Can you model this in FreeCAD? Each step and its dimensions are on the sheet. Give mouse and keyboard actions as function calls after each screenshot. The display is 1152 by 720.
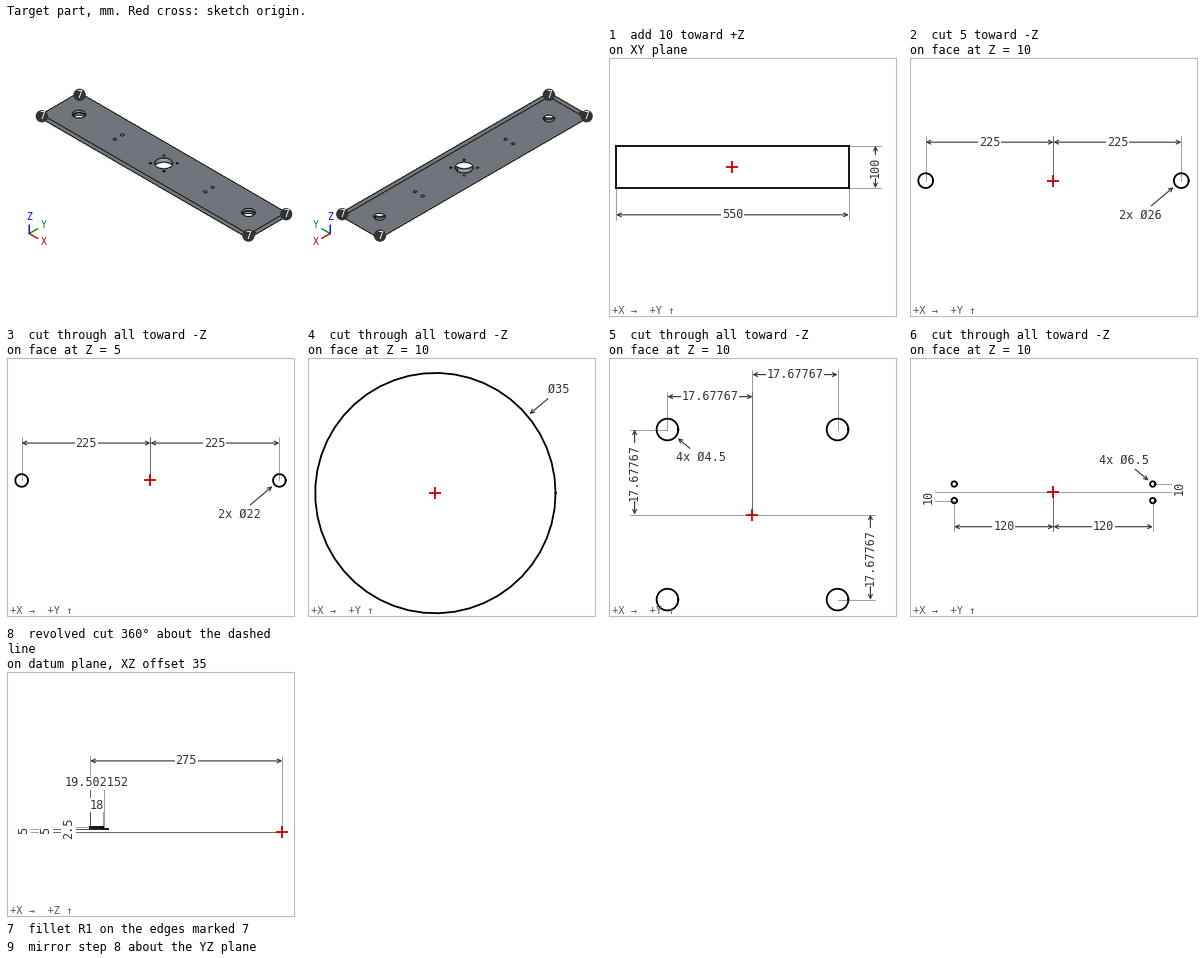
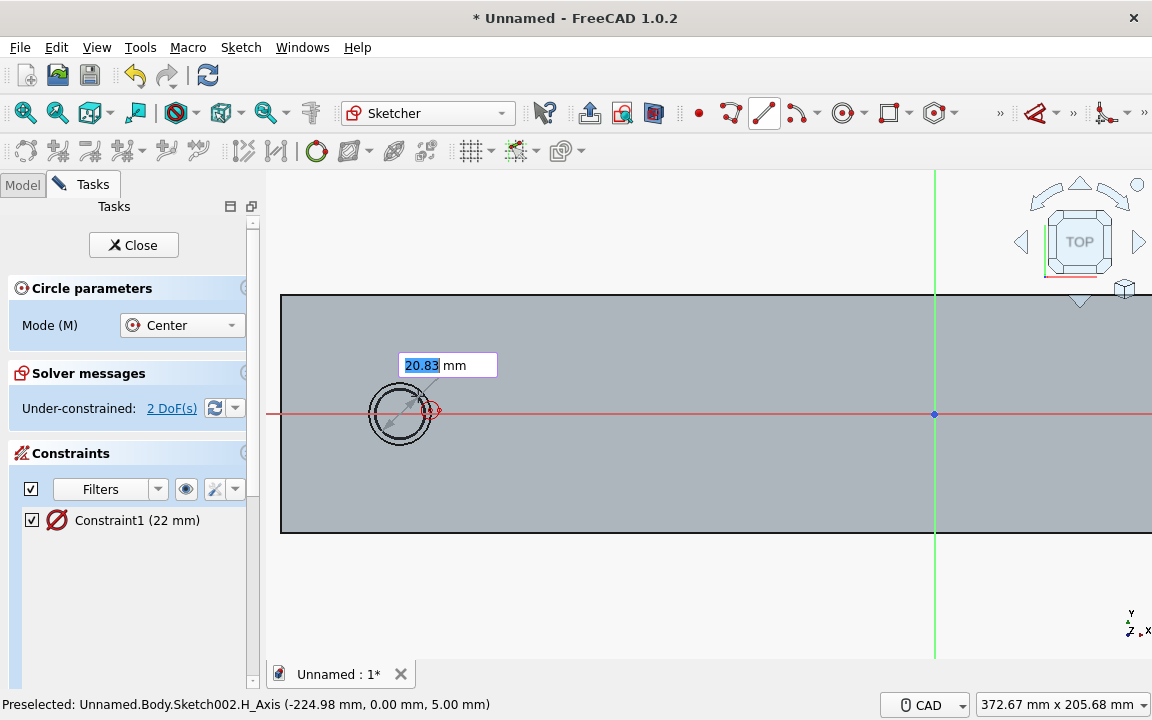
text(22)
key(Return)
key(Escape)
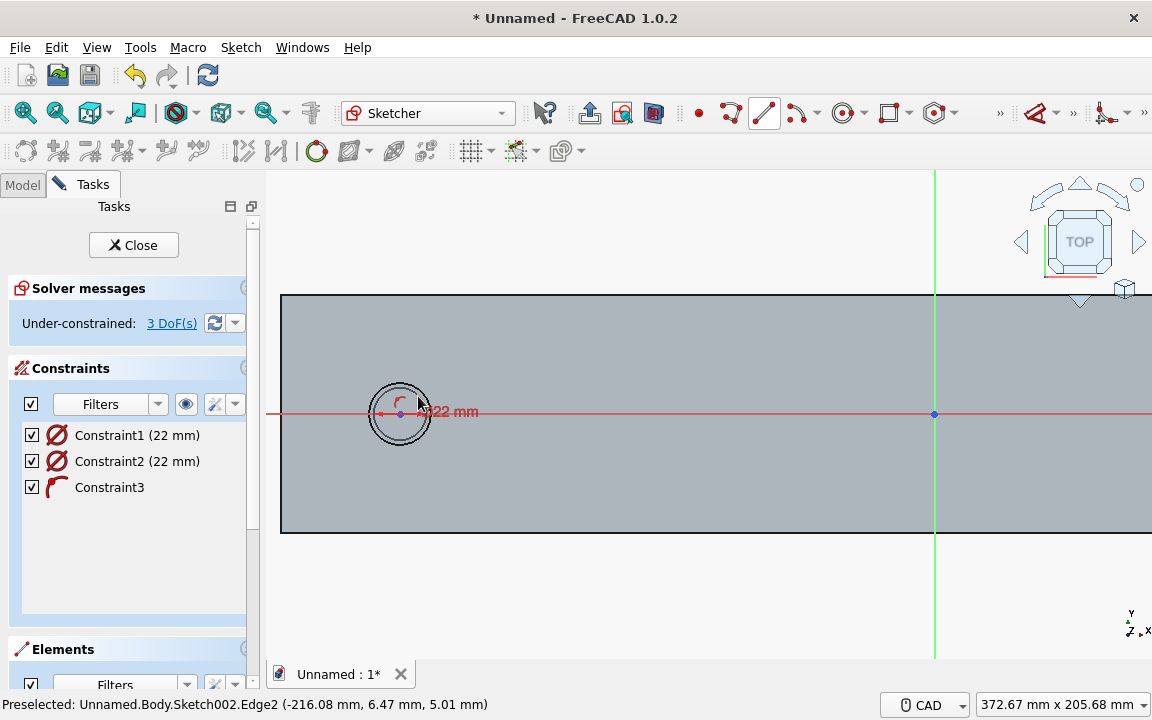
scroll(400, 415, down, 4)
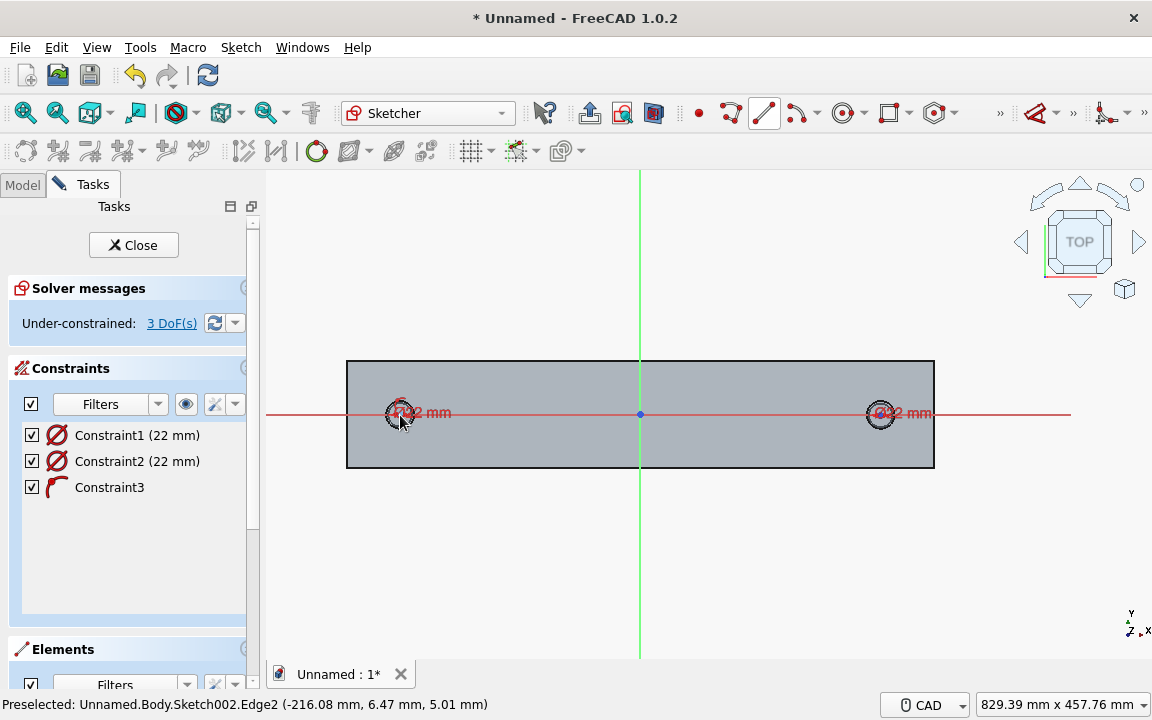
click(881, 415)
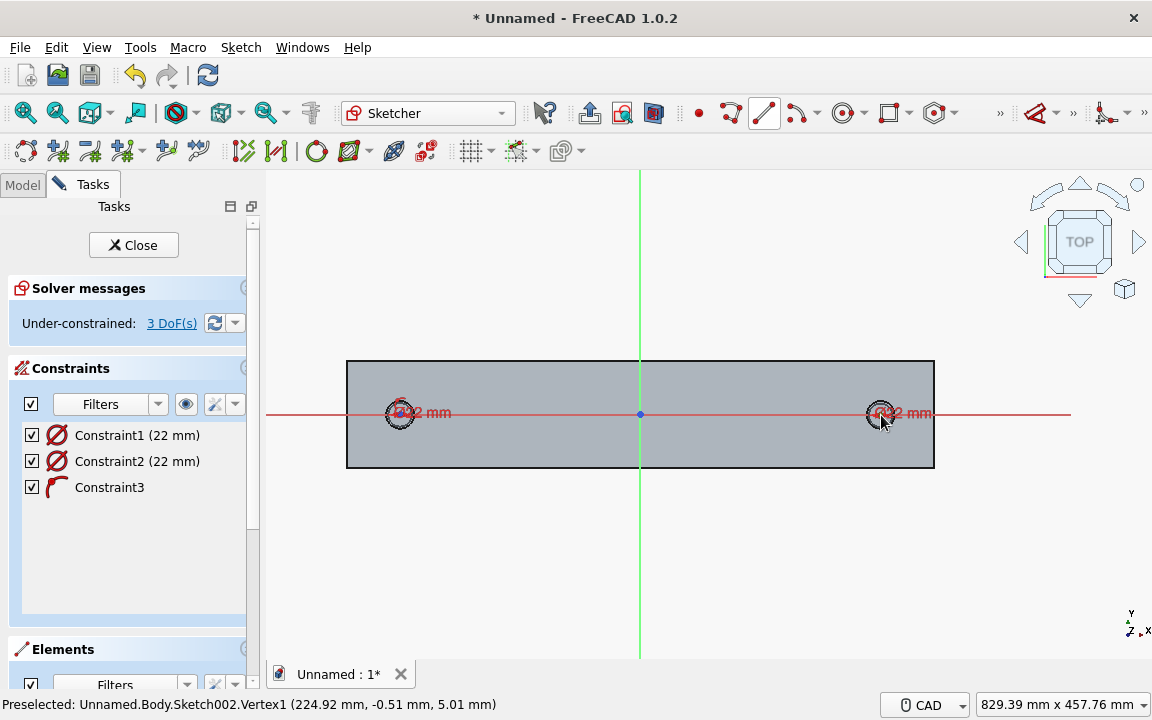
click(344, 415)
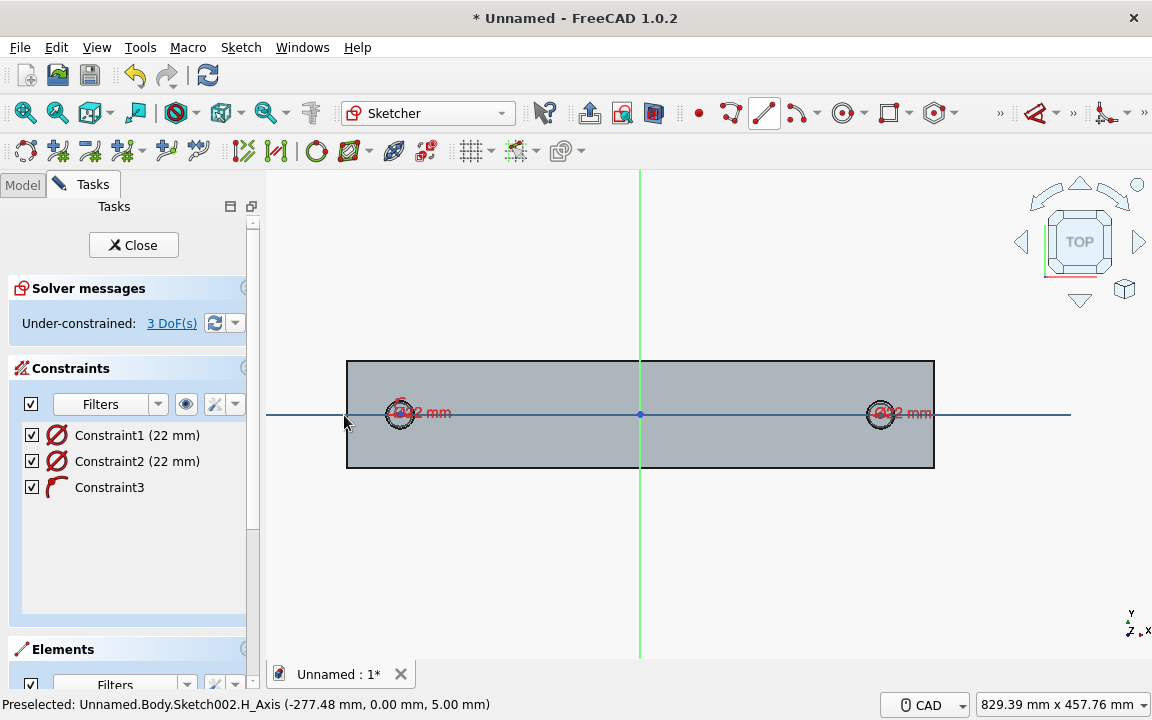
key(c)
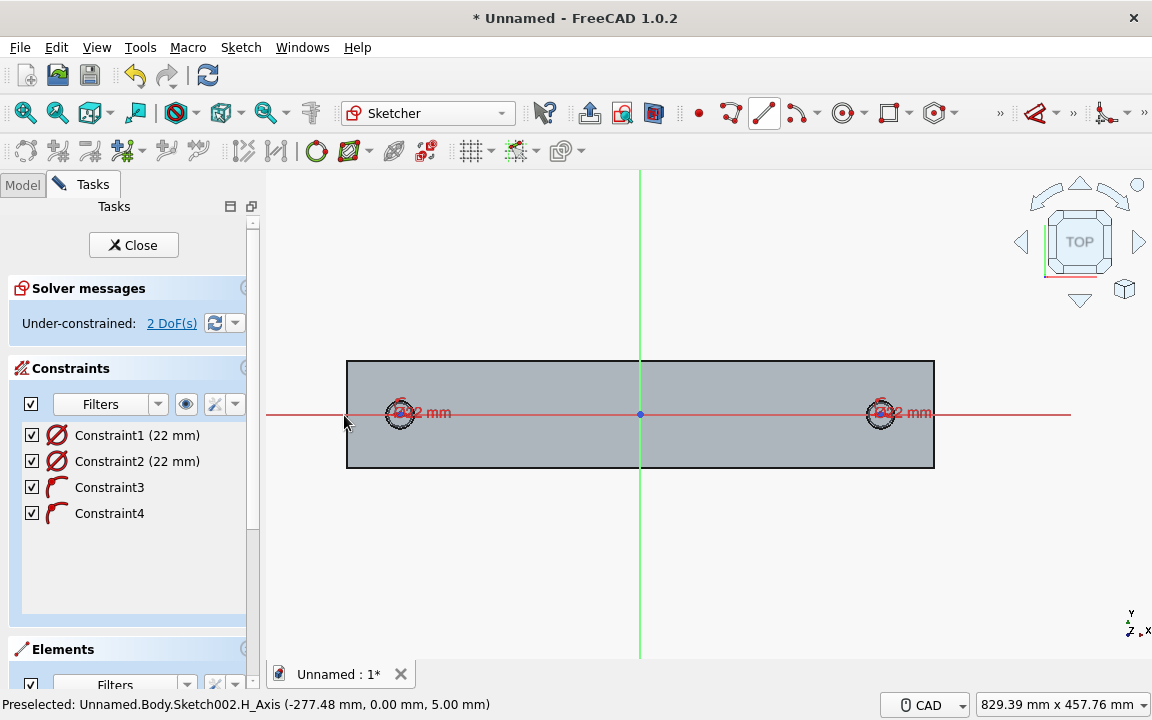
click(1036, 114)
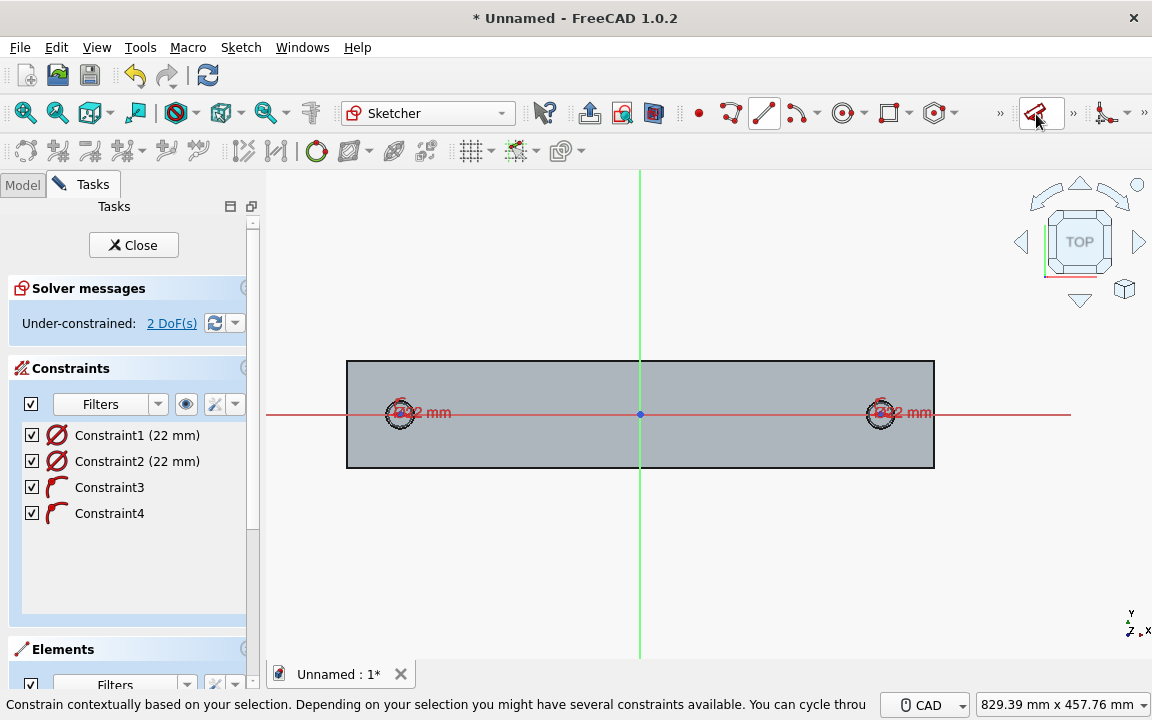
click(881, 415)
click(761, 449)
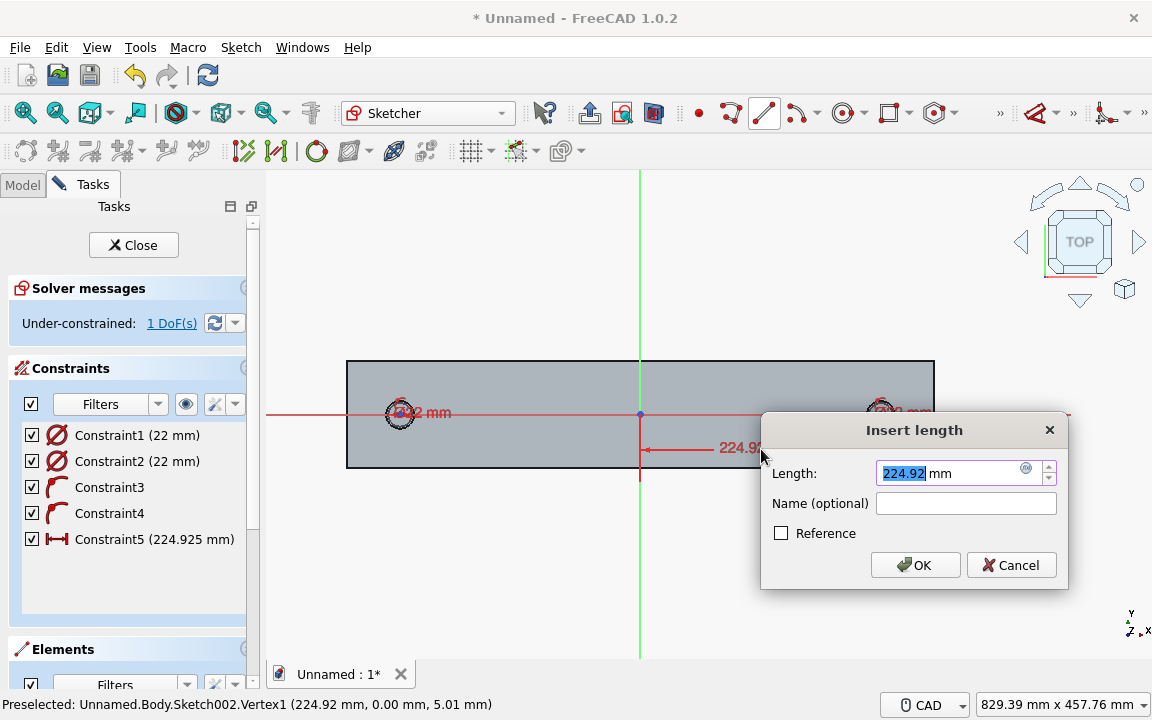
text(225)
key(Return)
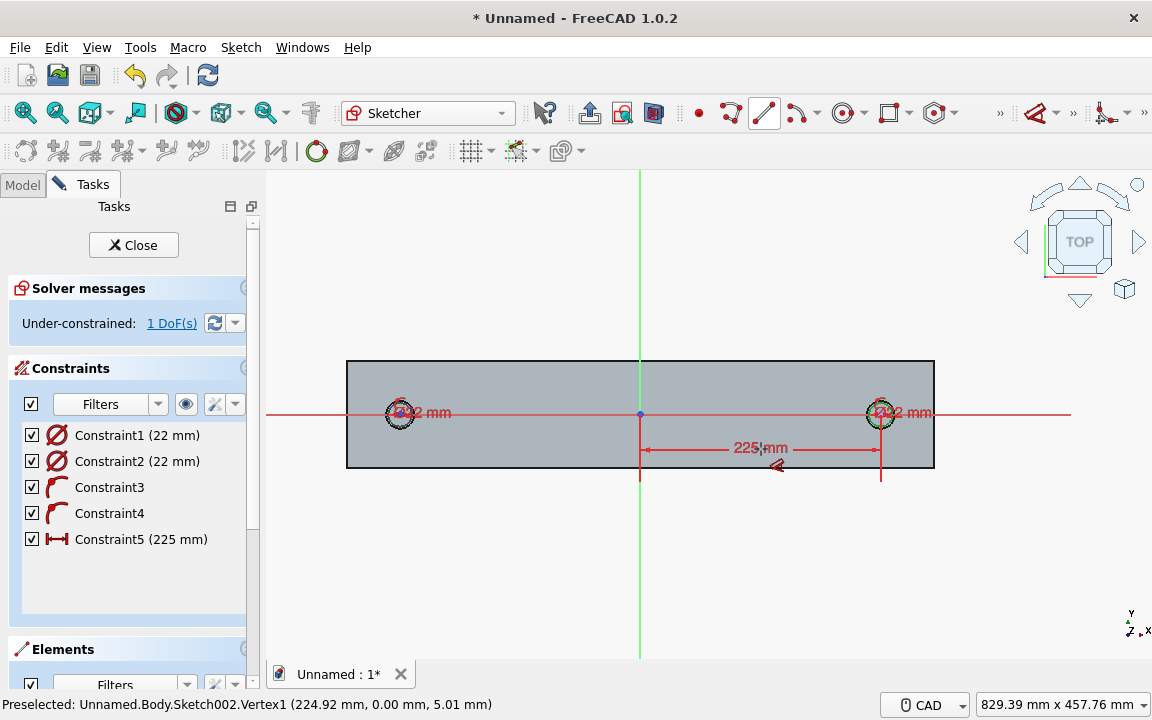
click(400, 415)
click(520, 449)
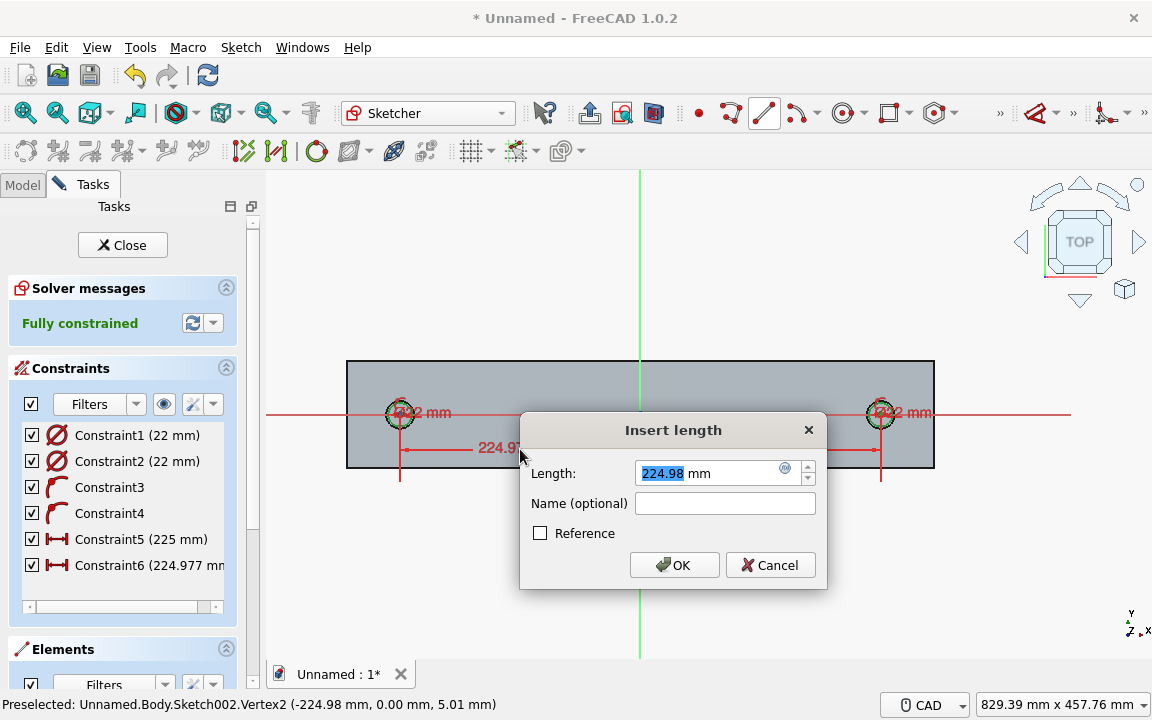
text(225)
key(Return)
key(Escape)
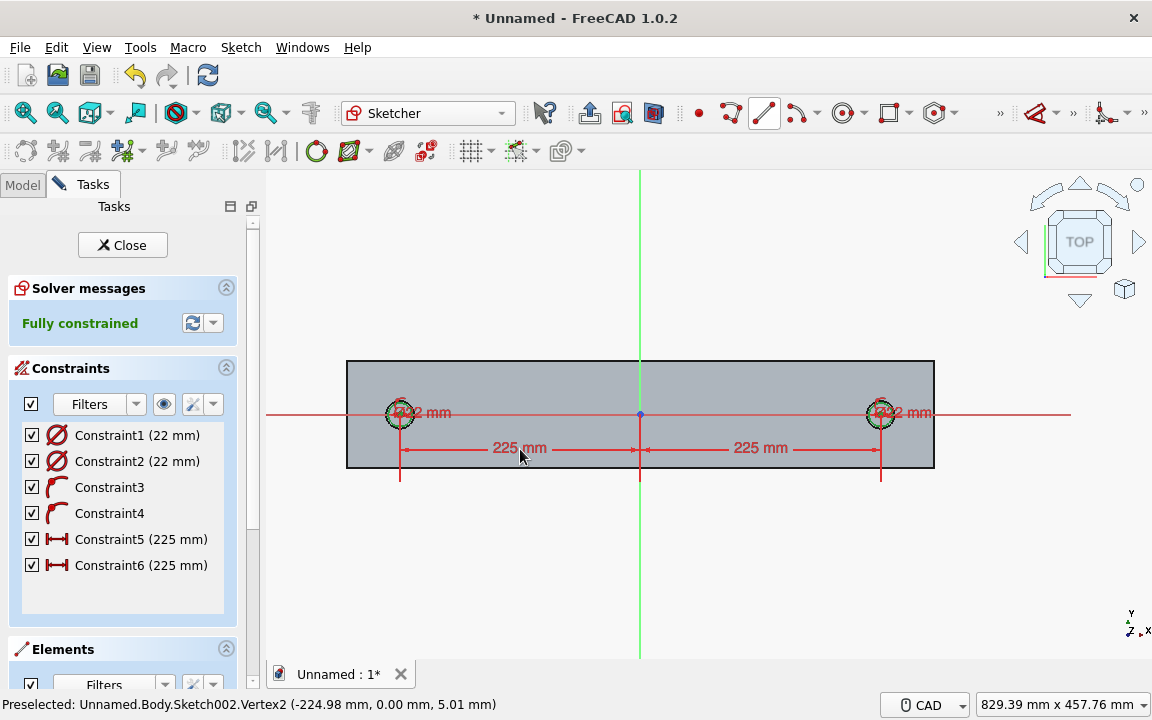
click(123, 245)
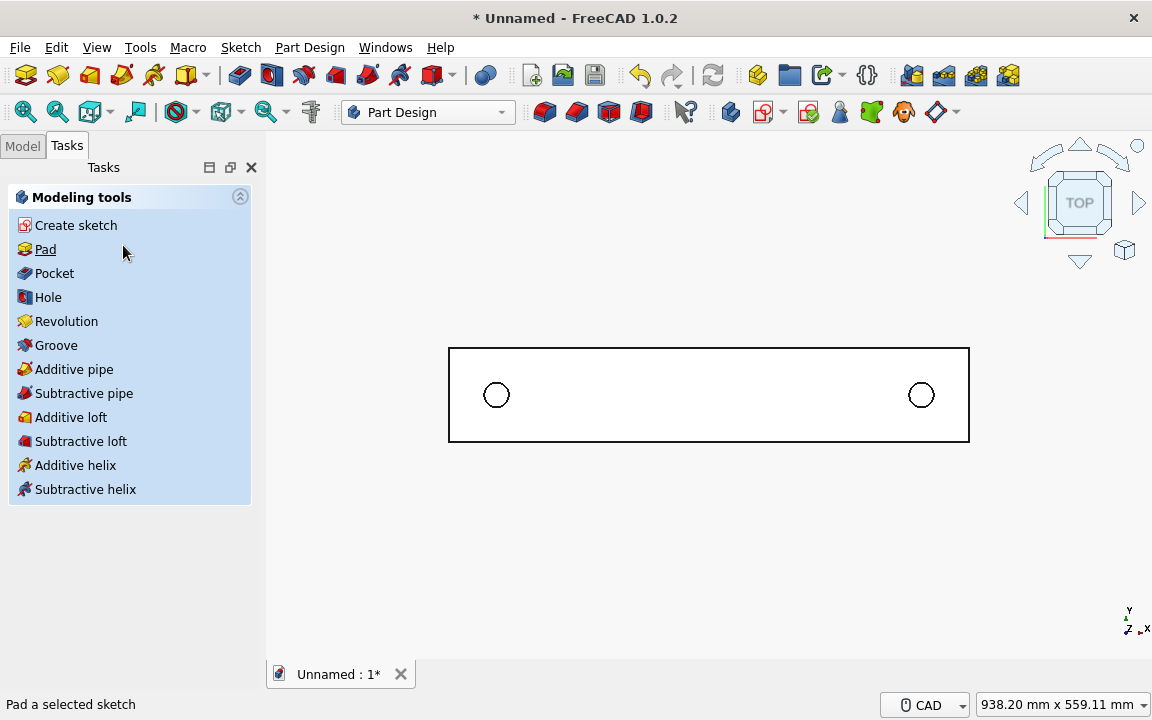
click(240, 76)